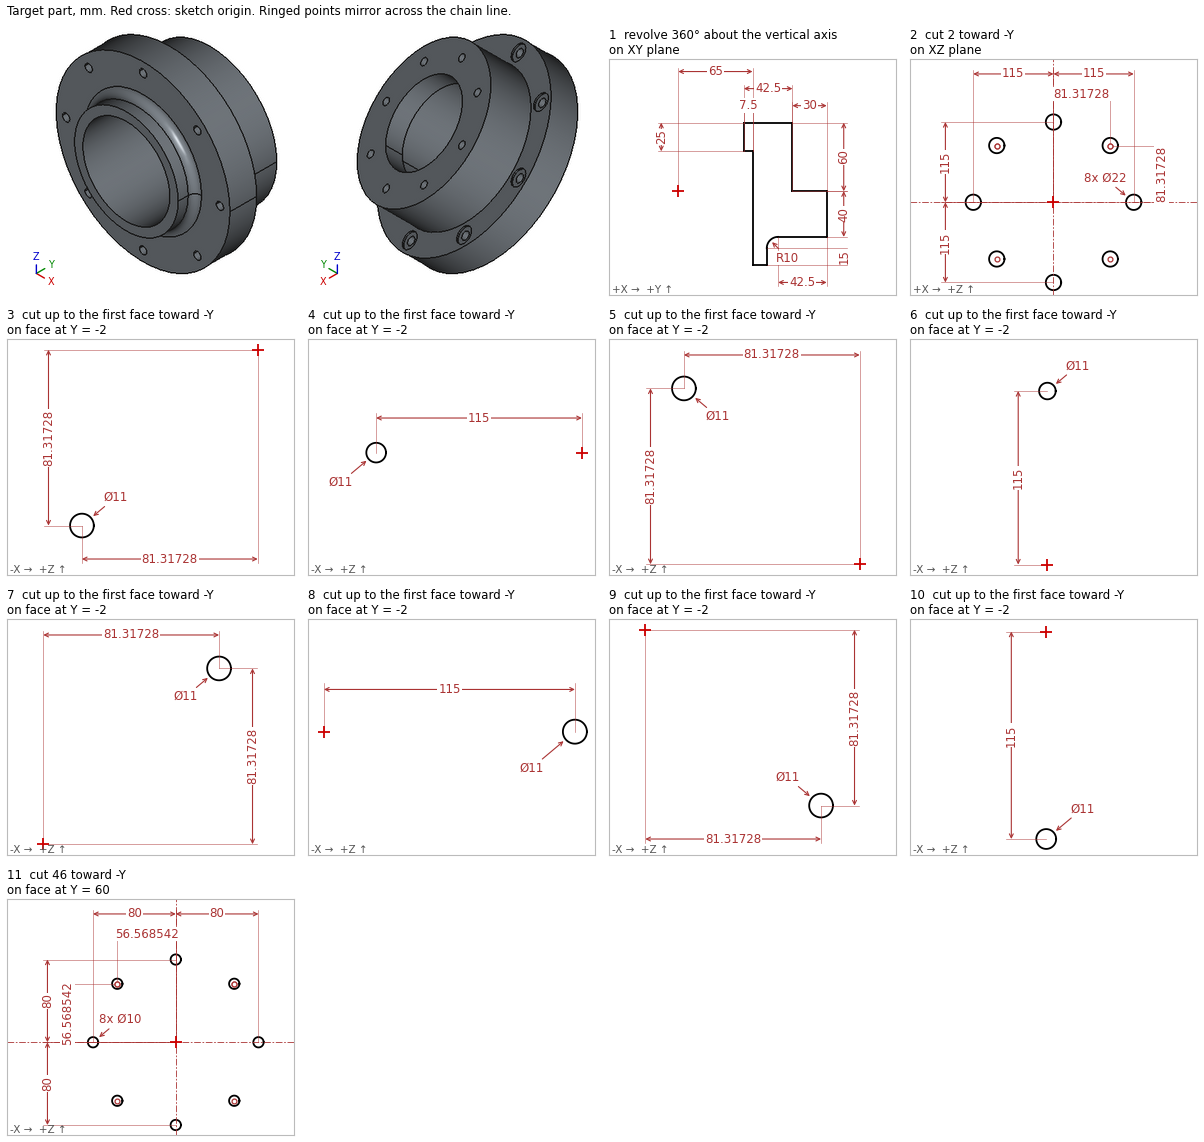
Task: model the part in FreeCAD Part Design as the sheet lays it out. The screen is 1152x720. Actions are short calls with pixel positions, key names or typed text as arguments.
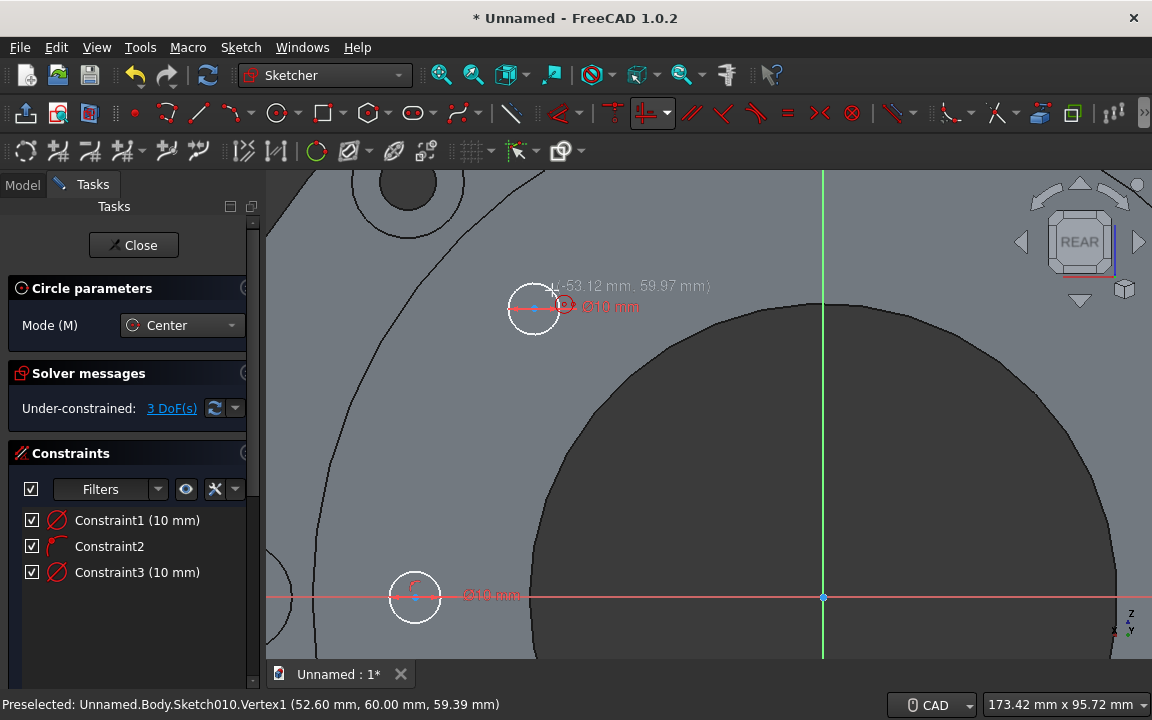
scroll(534, 308, down, 5)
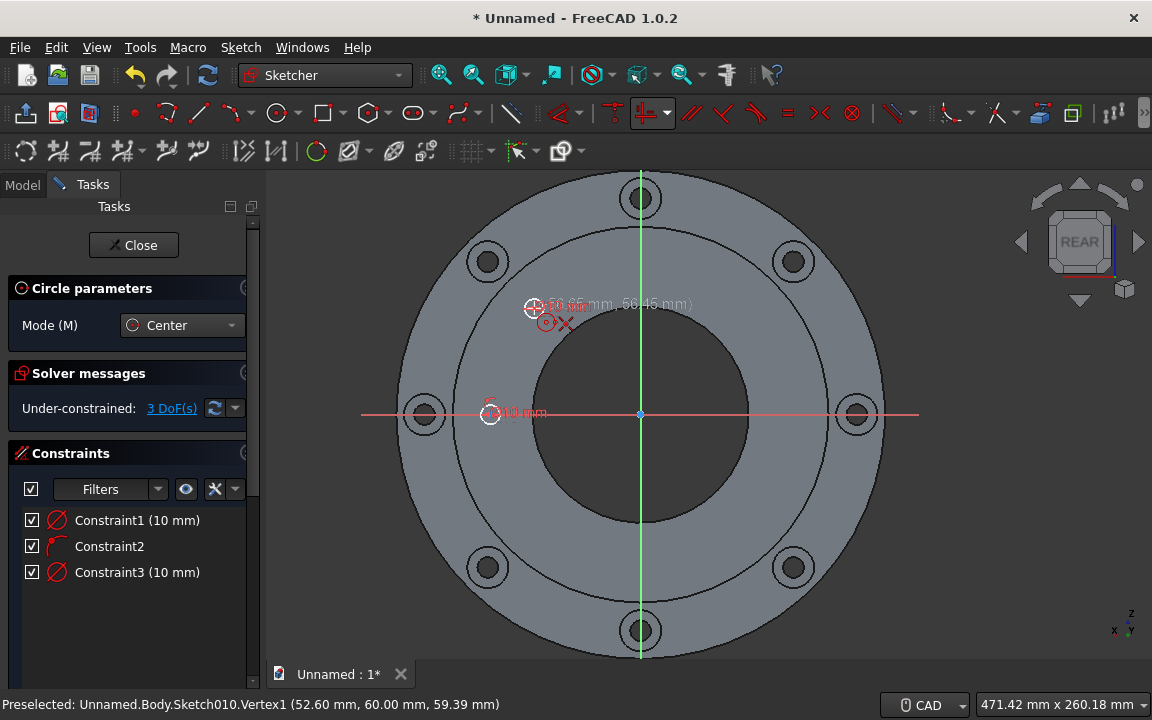
scroll(641, 264, up, 5)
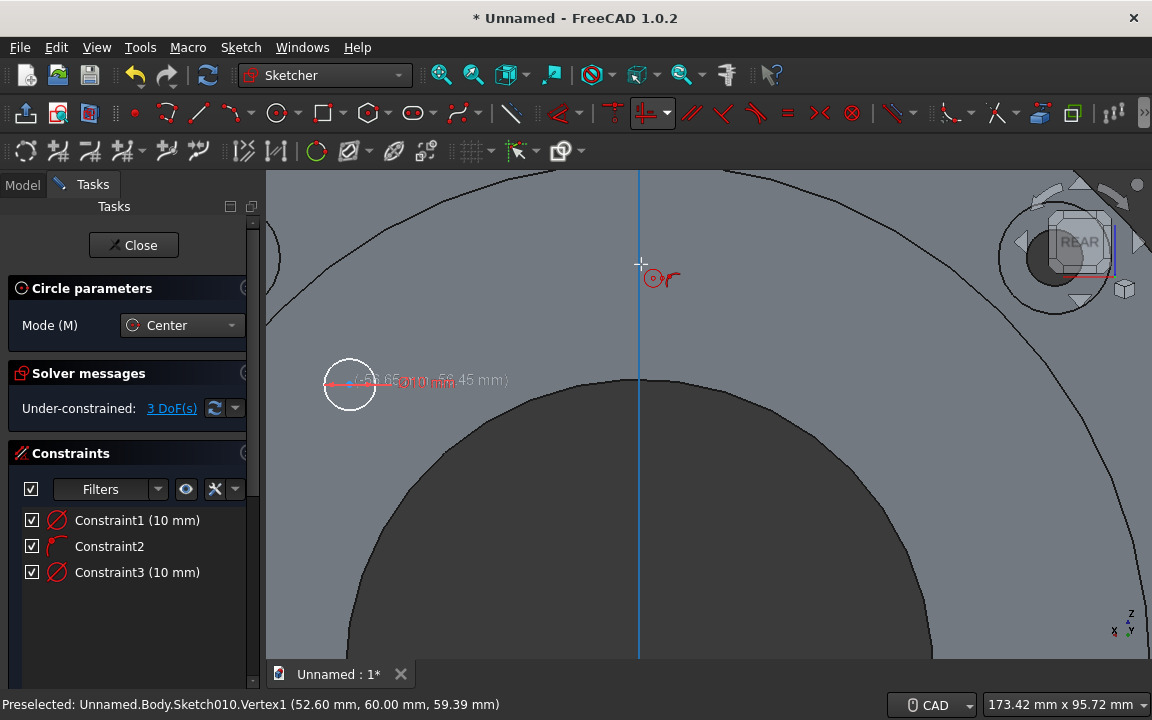
click(639, 264)
move(657, 246)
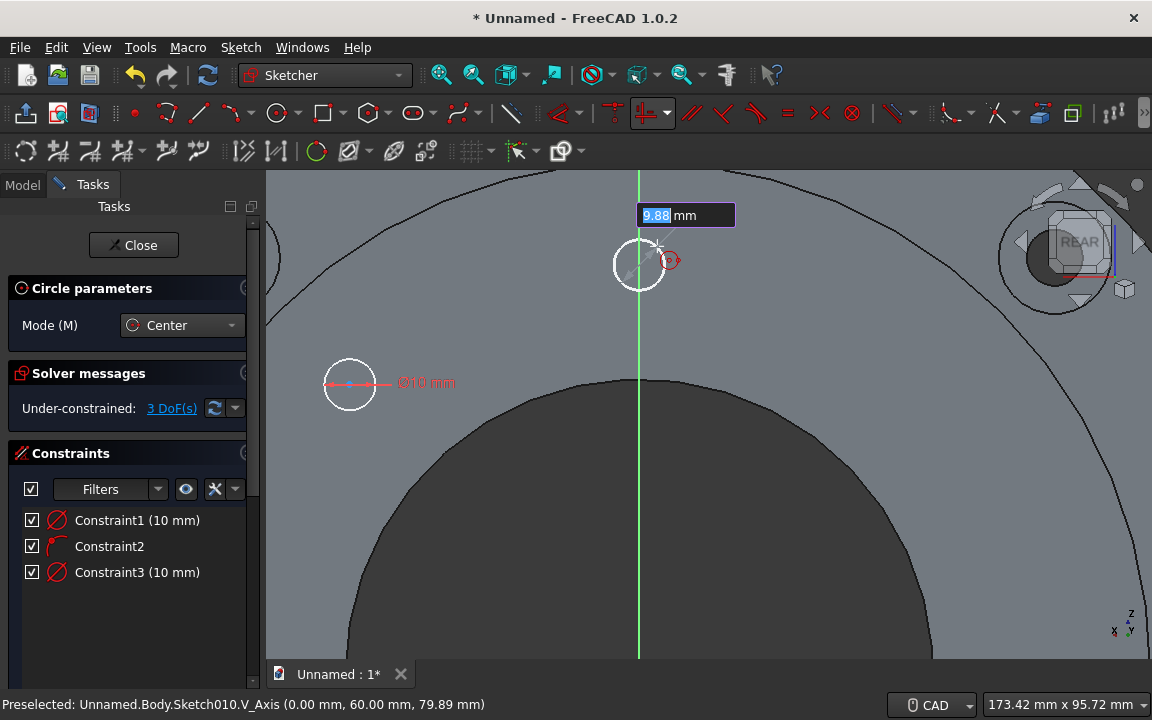
text(10)
key(Return)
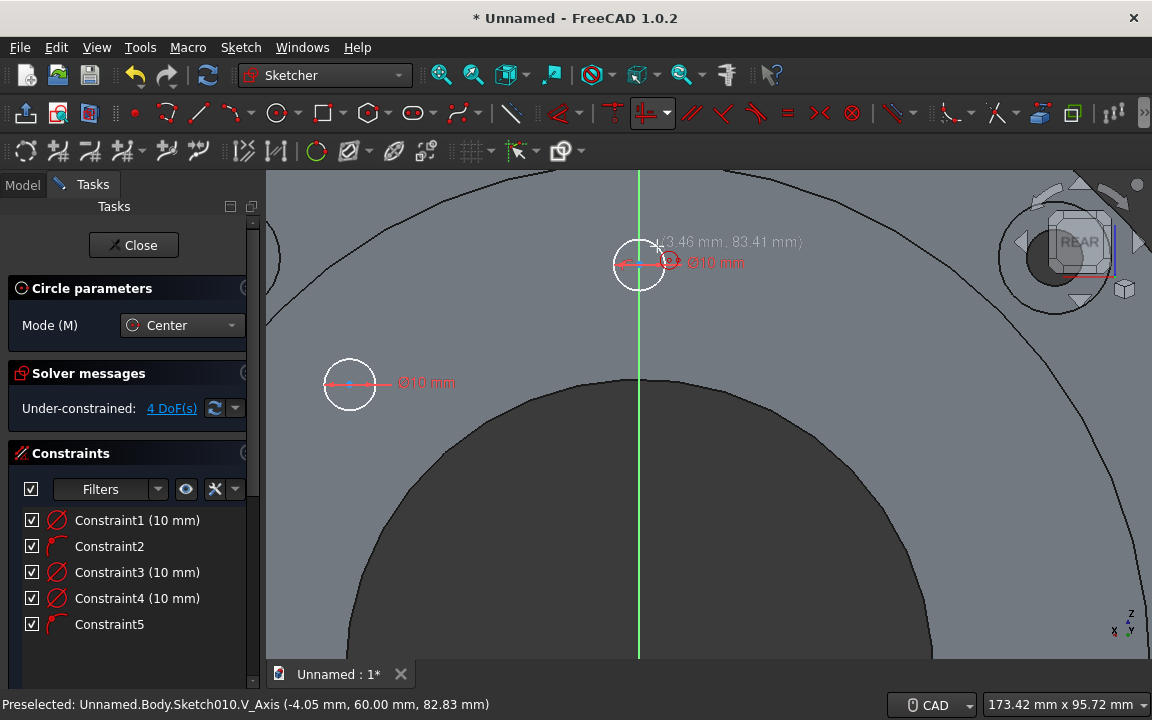
click(928, 384)
move(946, 366)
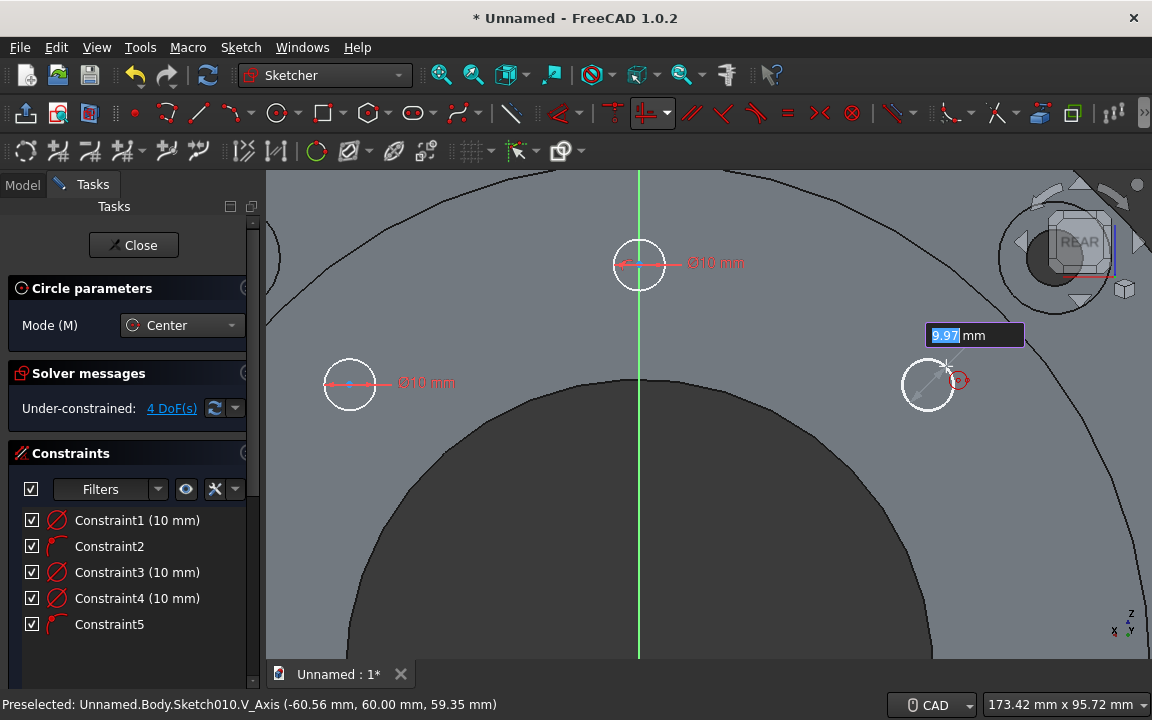
text(10)
key(Return)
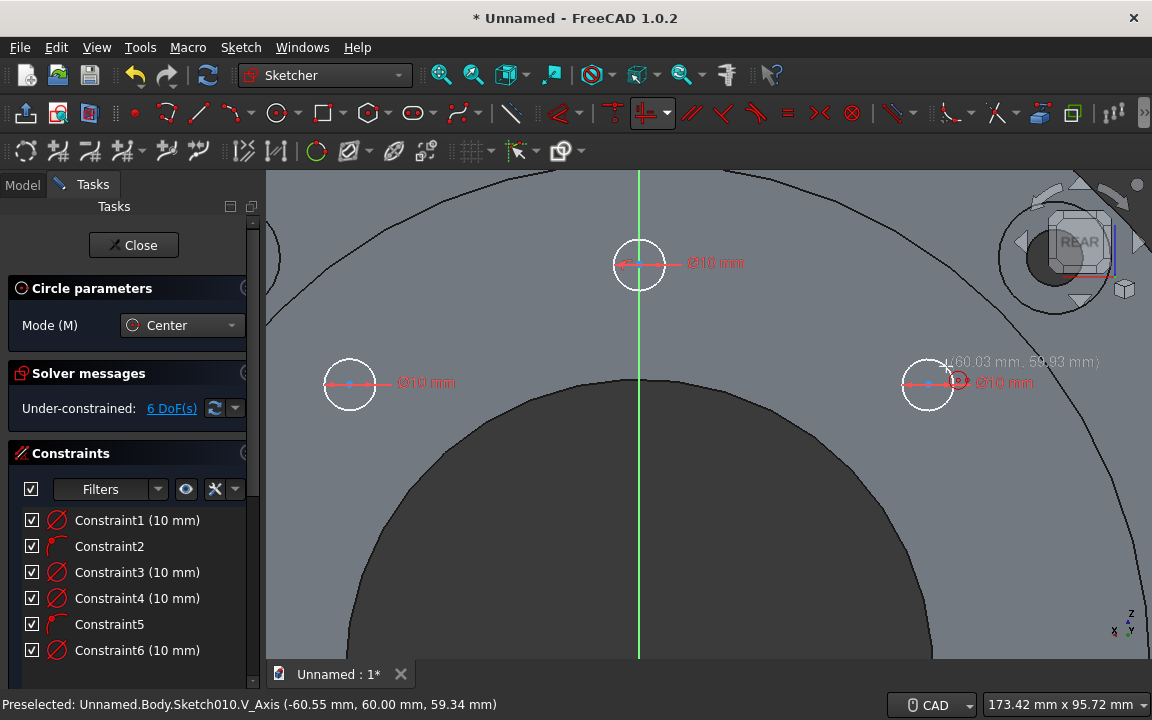
scroll(641, 264, down, 5)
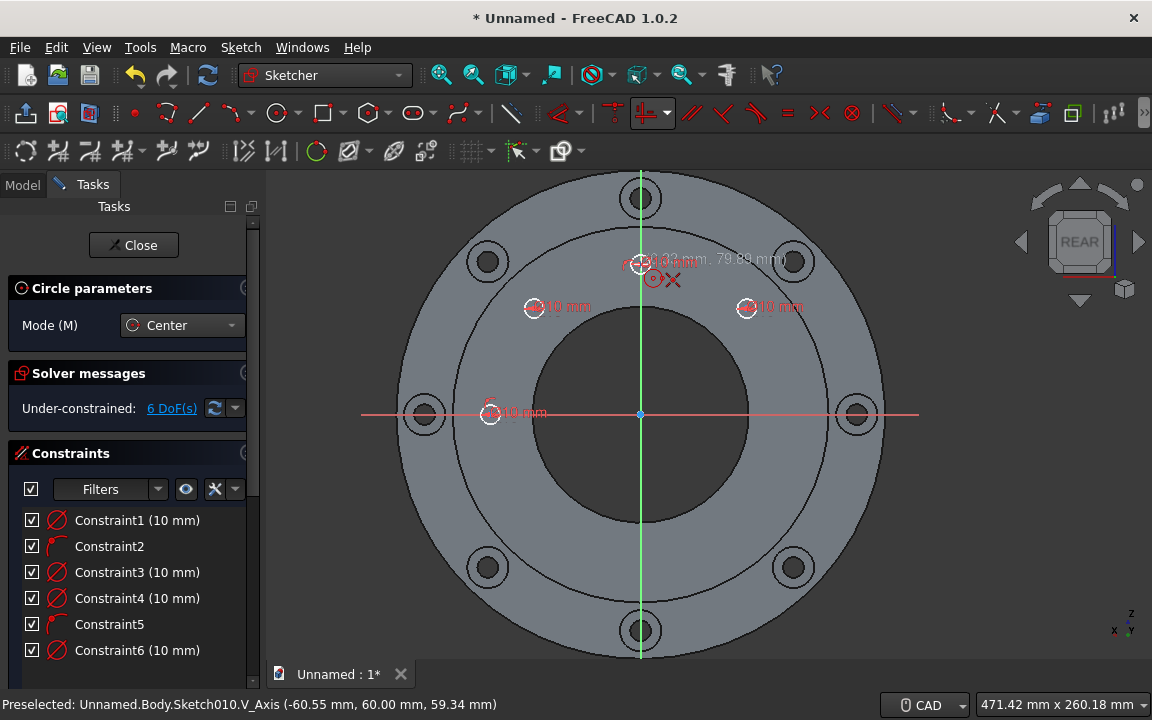
scroll(791, 415, up, 5)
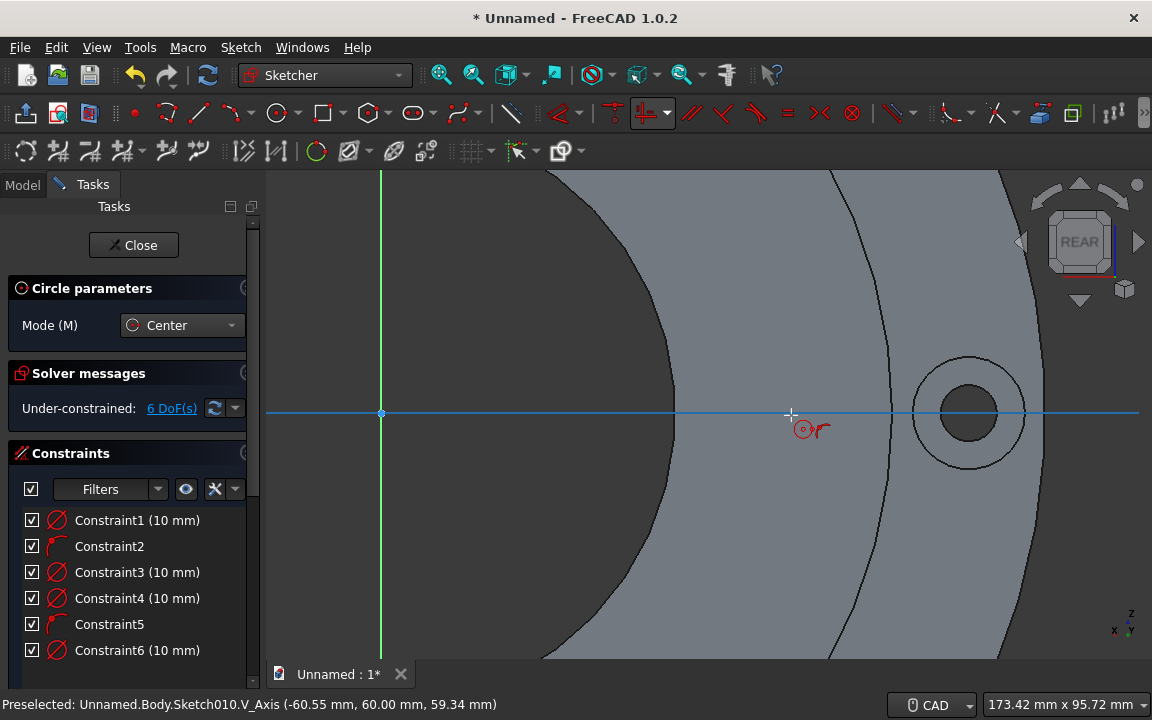
click(790, 413)
move(808, 395)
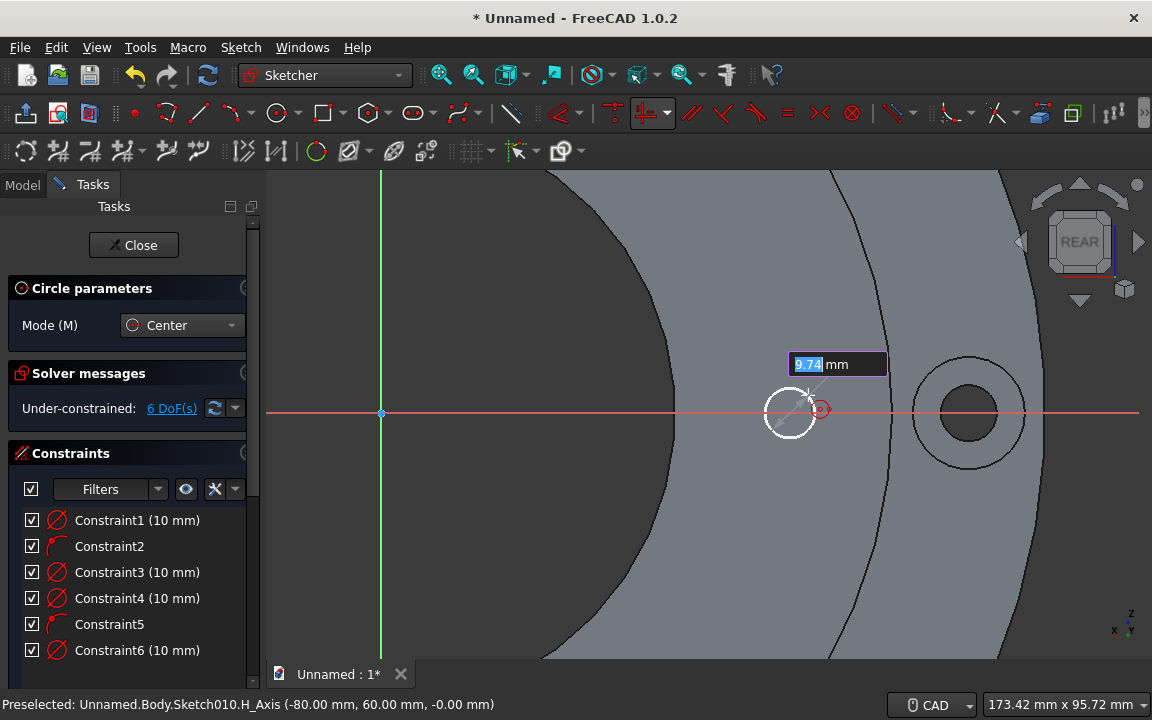
text(10)
key(Return)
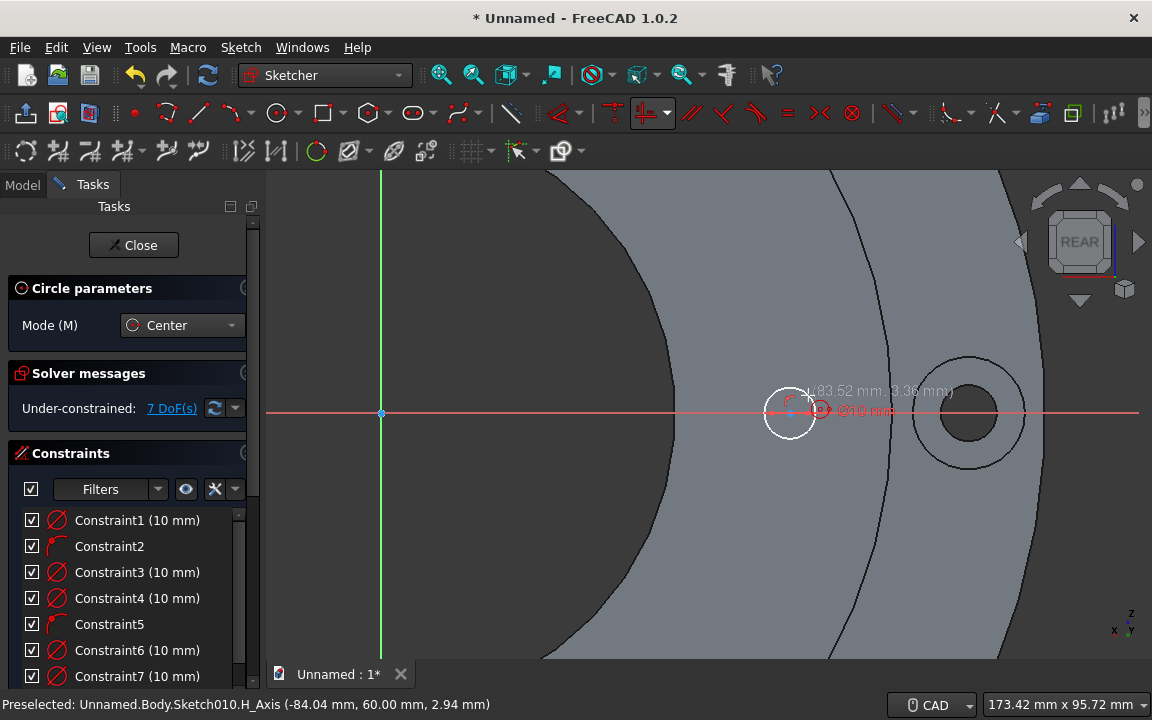
scroll(791, 415, down, 5)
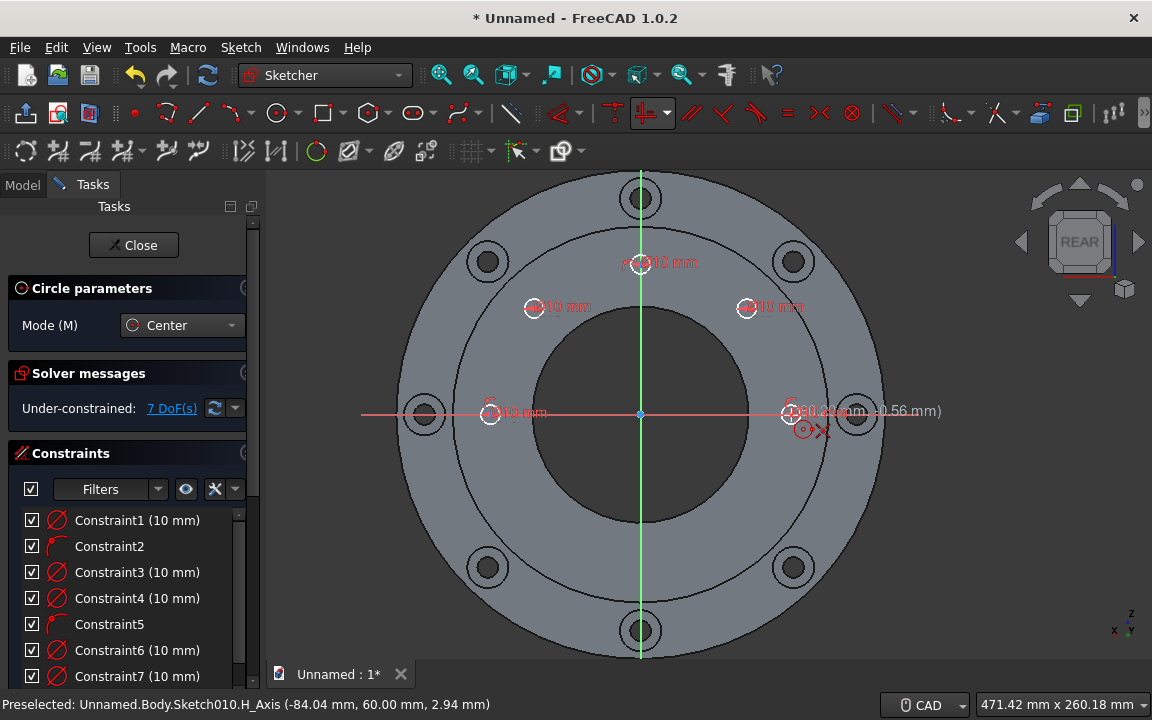
scroll(747, 521, up, 5)